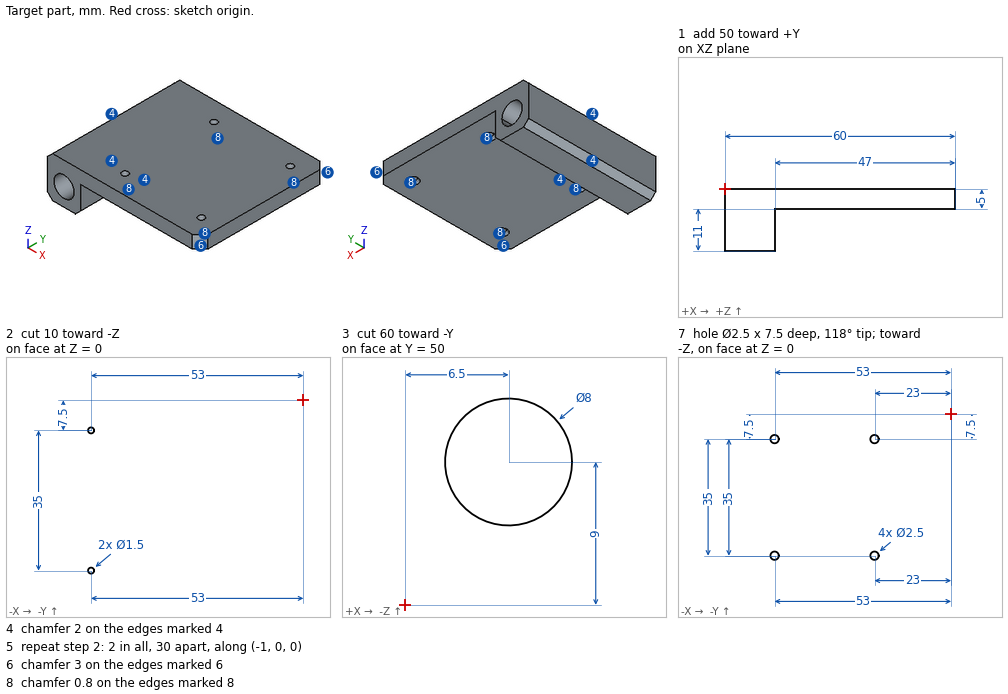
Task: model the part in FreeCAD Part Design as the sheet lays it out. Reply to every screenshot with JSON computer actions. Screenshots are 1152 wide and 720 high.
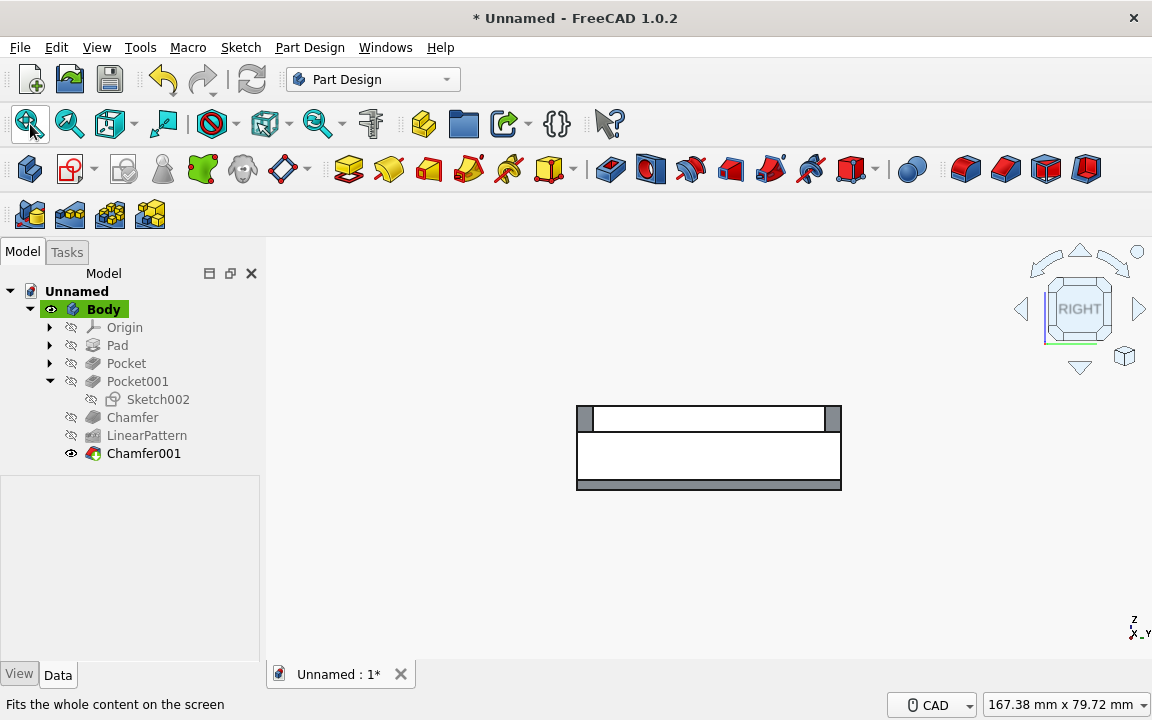
{"action": "key", "text": "0"}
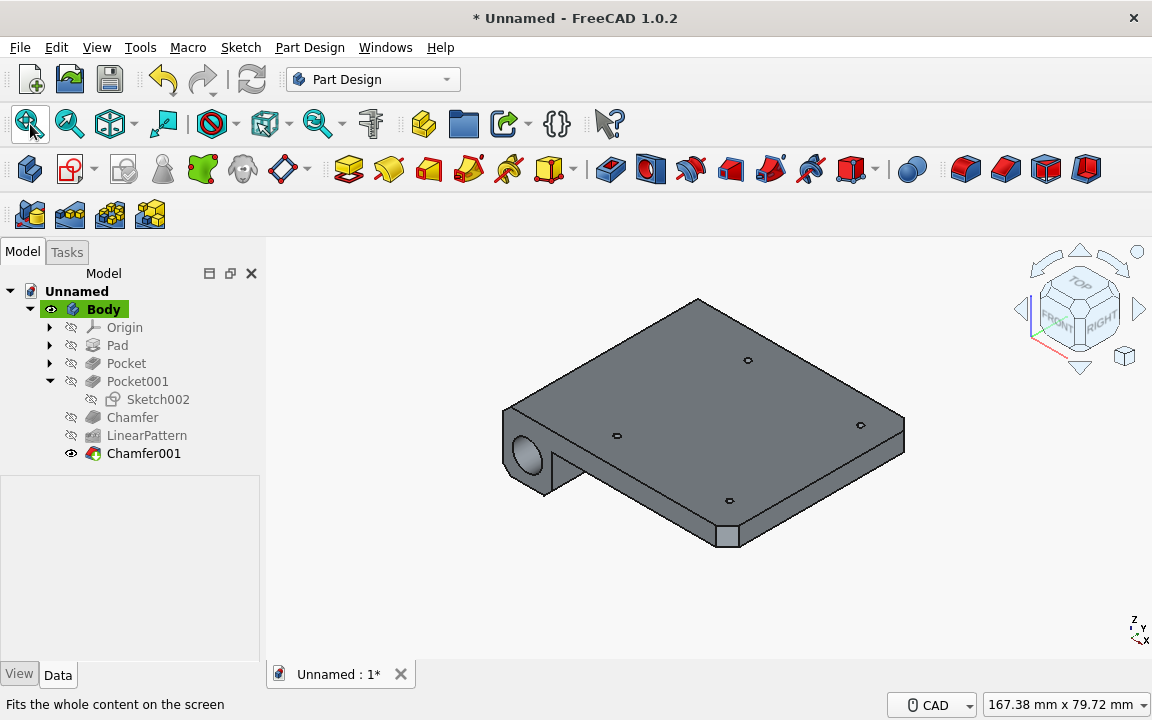
{"action": "left_click", "coordinate": [744, 432]}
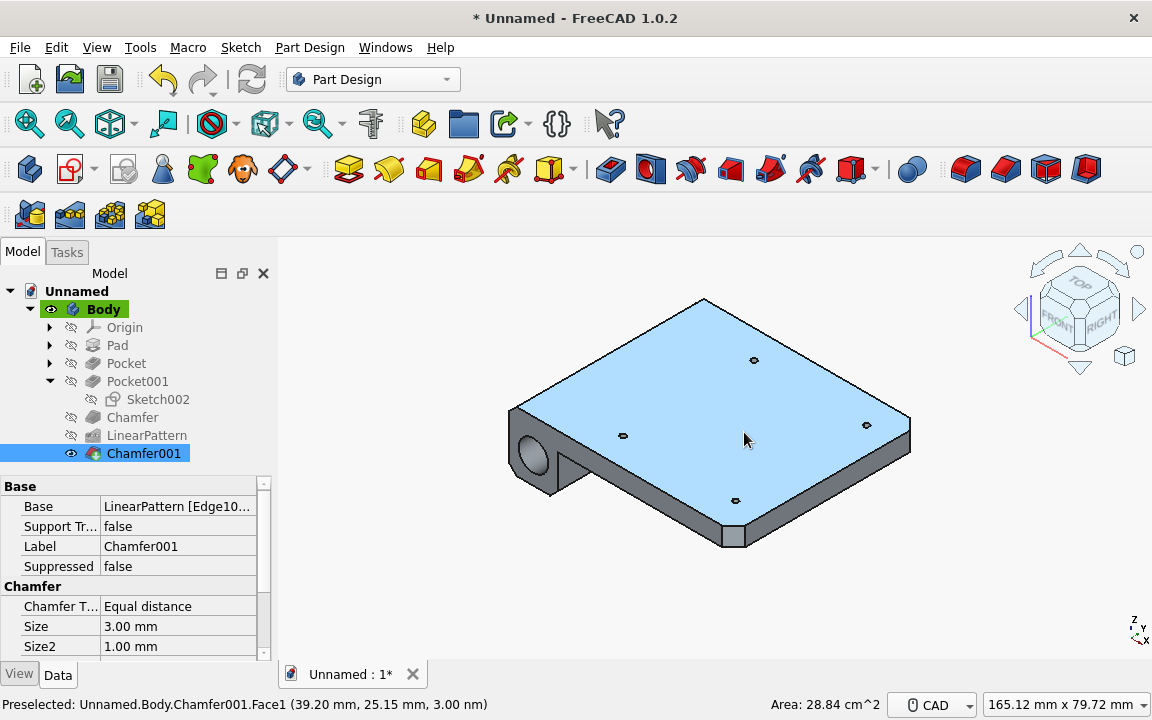
{"action": "left_click", "coordinate": [70, 170]}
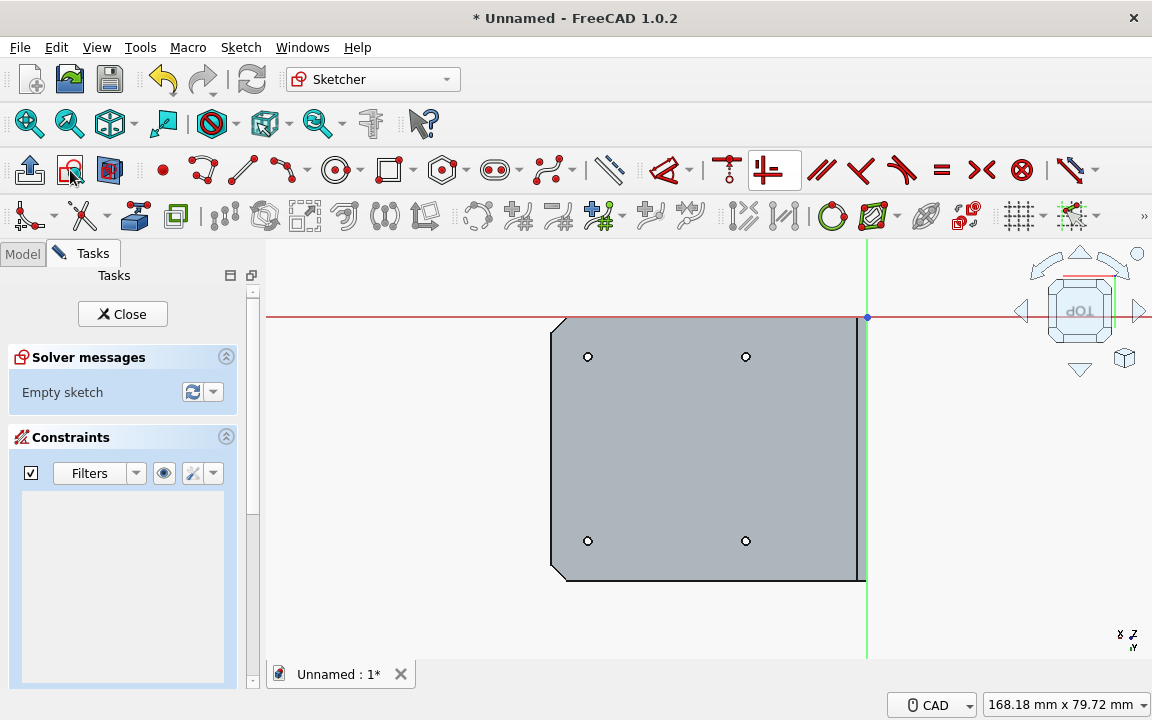
{"action": "left_click", "coordinate": [336, 170]}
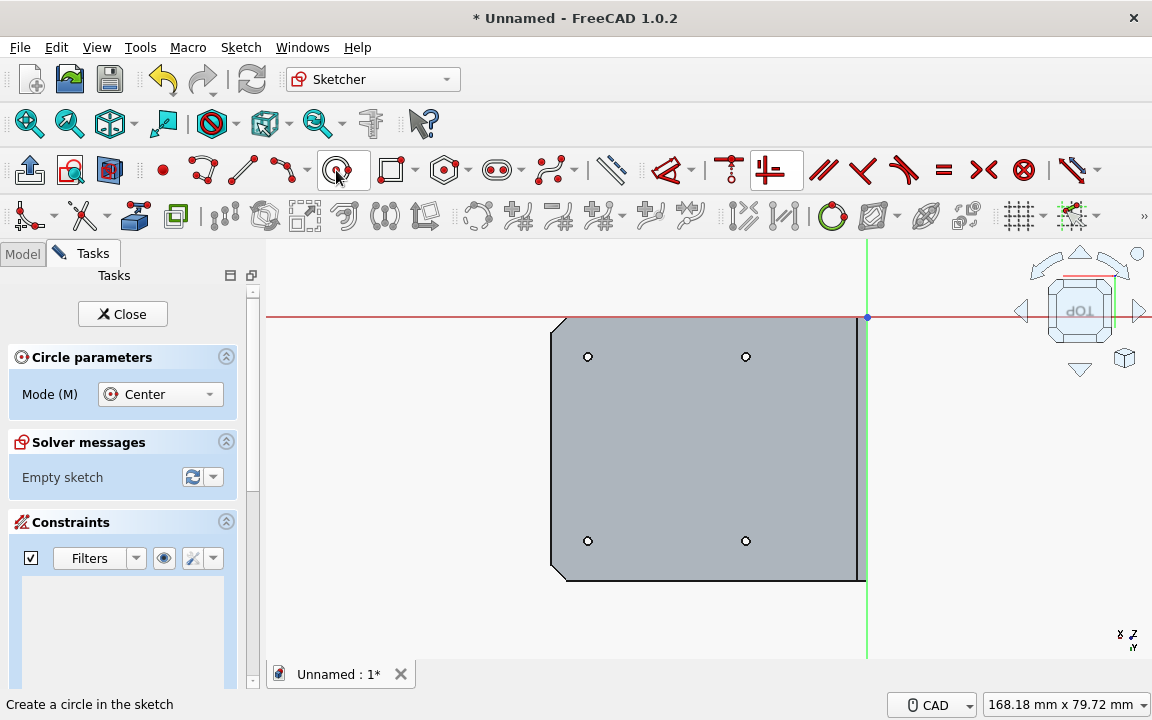
{"action": "scroll", "coordinate": [746, 541], "scroll_direction": "up", "scroll_amount": 7}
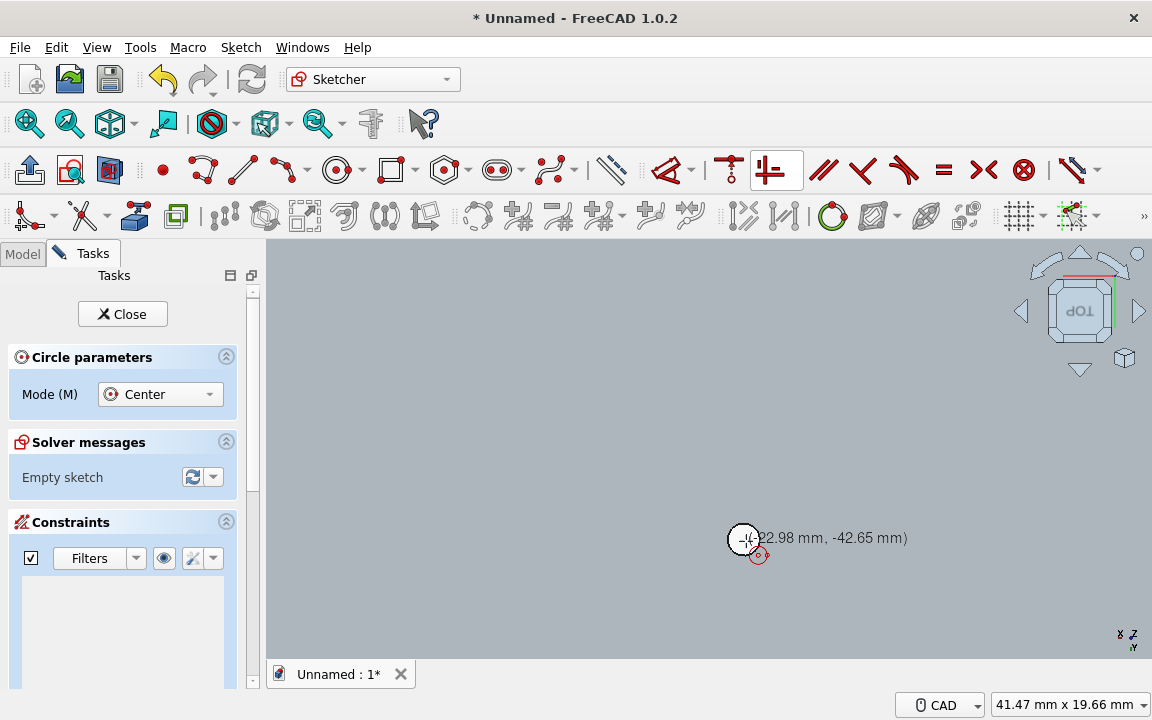
{"action": "scroll", "coordinate": [634, 600], "scroll_direction": "down", "scroll_amount": 6}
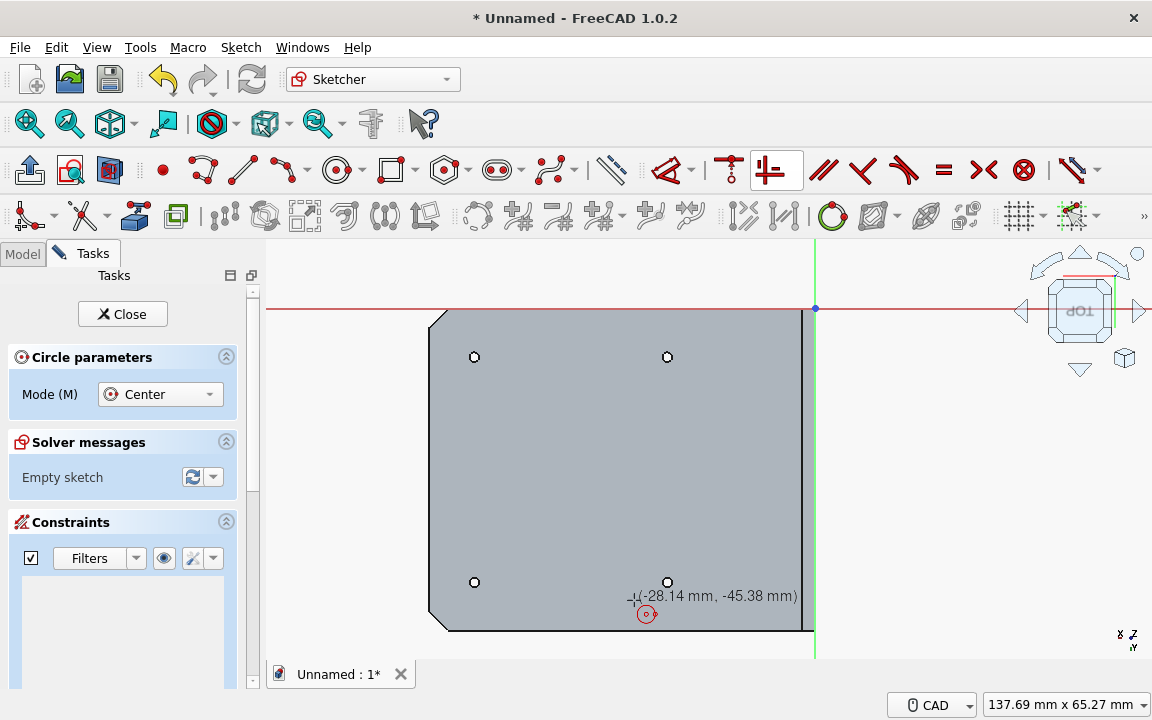
{"action": "left_click", "coordinate": [667, 582]}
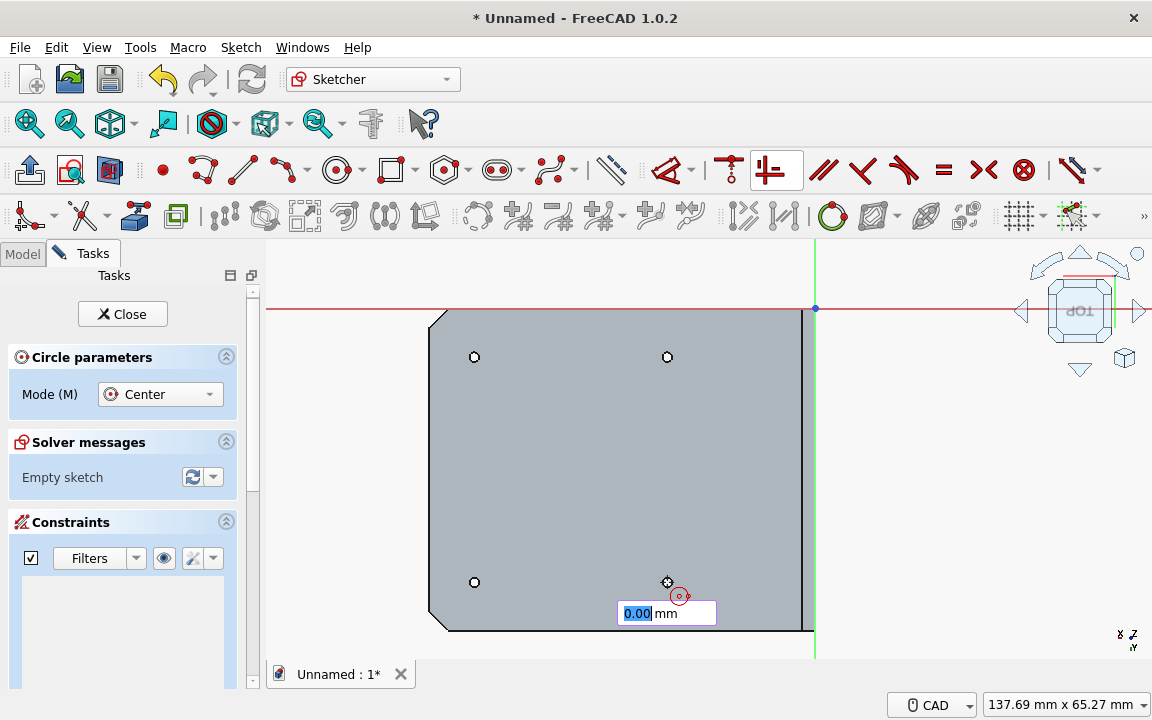
{"action": "scroll", "coordinate": [673, 577], "scroll_direction": "up", "scroll_amount": 4}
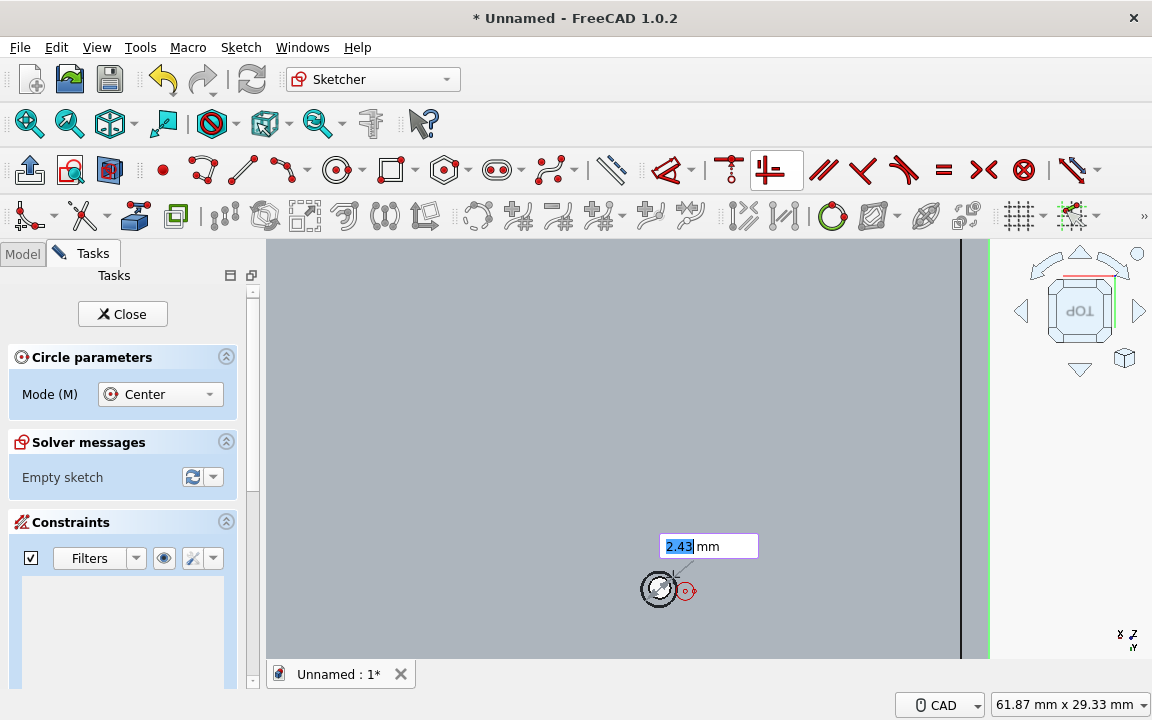
{"action": "left_click", "coordinate": [673, 575]}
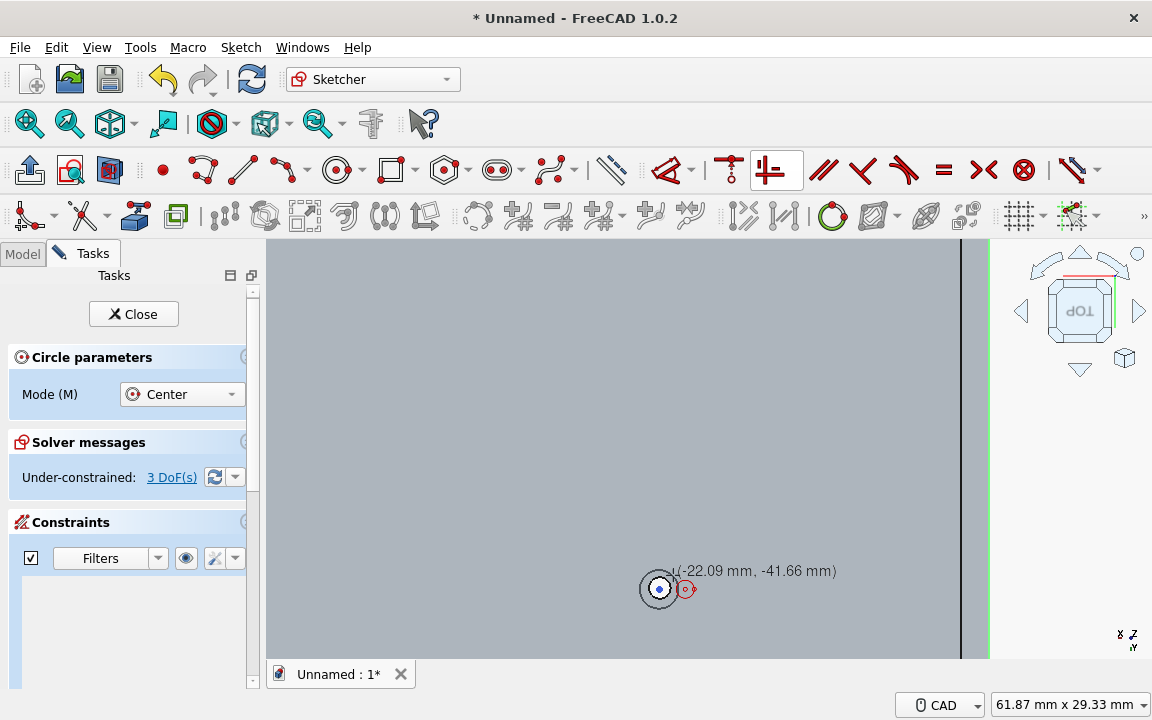
{"action": "scroll", "coordinate": [673, 577], "scroll_direction": "down", "scroll_amount": 4}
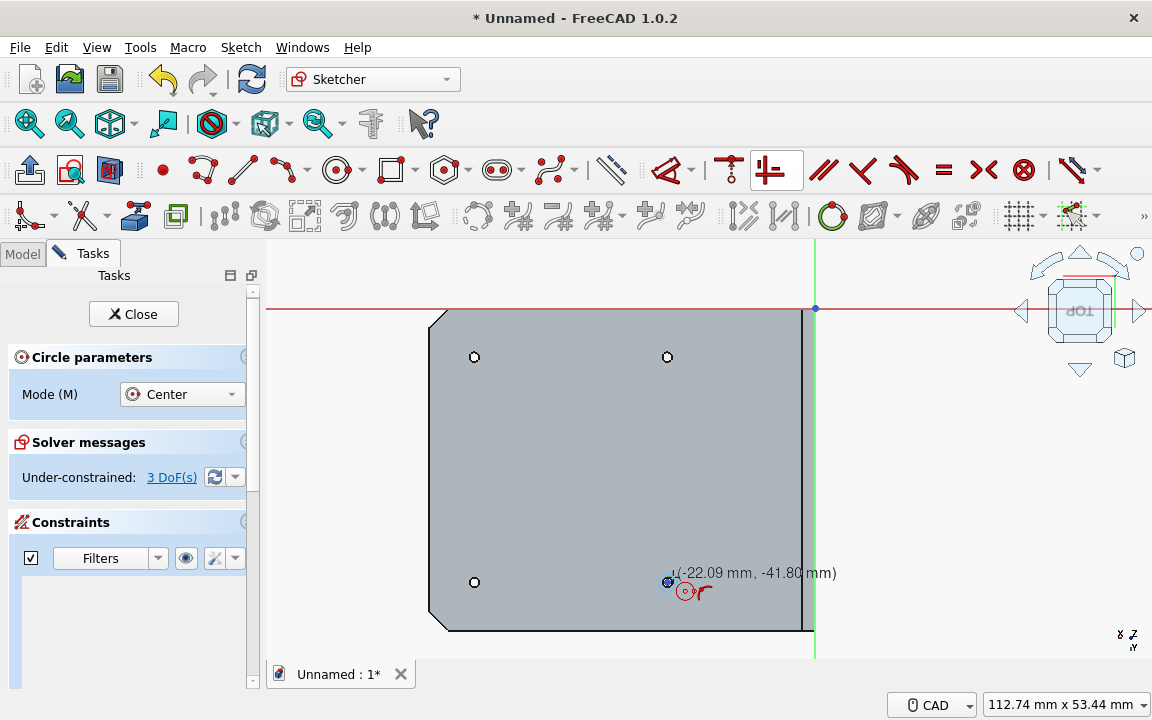
{"action": "scroll", "coordinate": [474, 582], "scroll_direction": "up", "scroll_amount": 6}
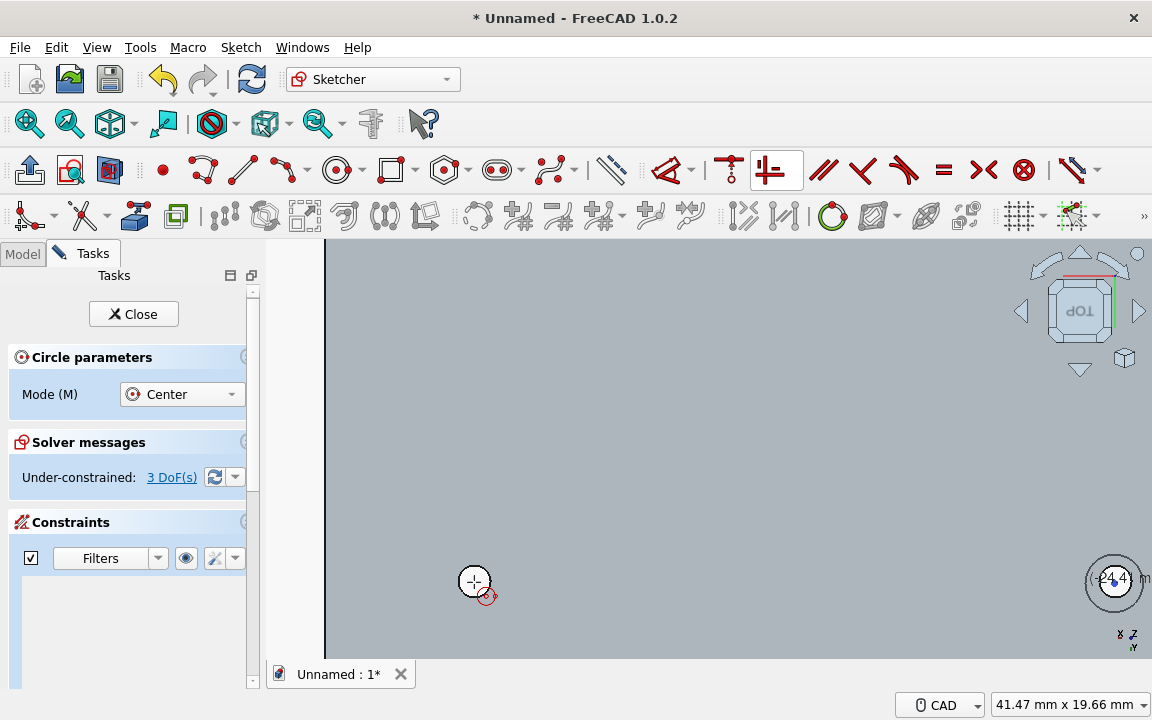
{"action": "scroll", "coordinate": [474, 582], "scroll_direction": "down", "scroll_amount": 6}